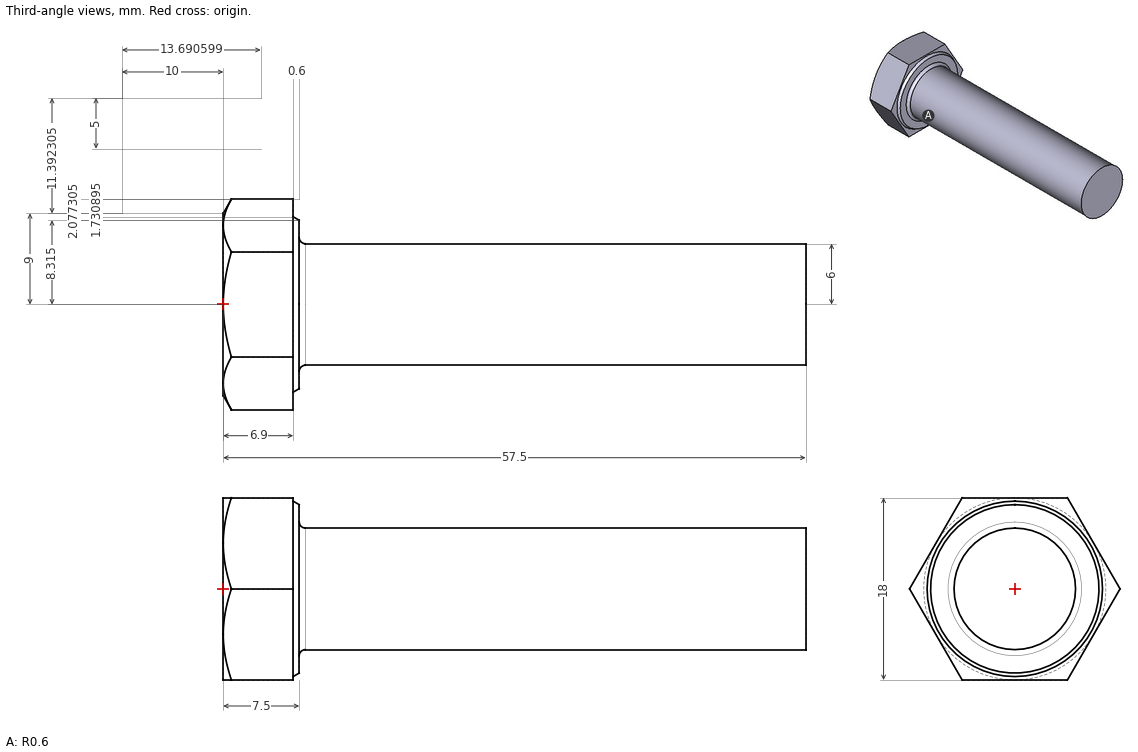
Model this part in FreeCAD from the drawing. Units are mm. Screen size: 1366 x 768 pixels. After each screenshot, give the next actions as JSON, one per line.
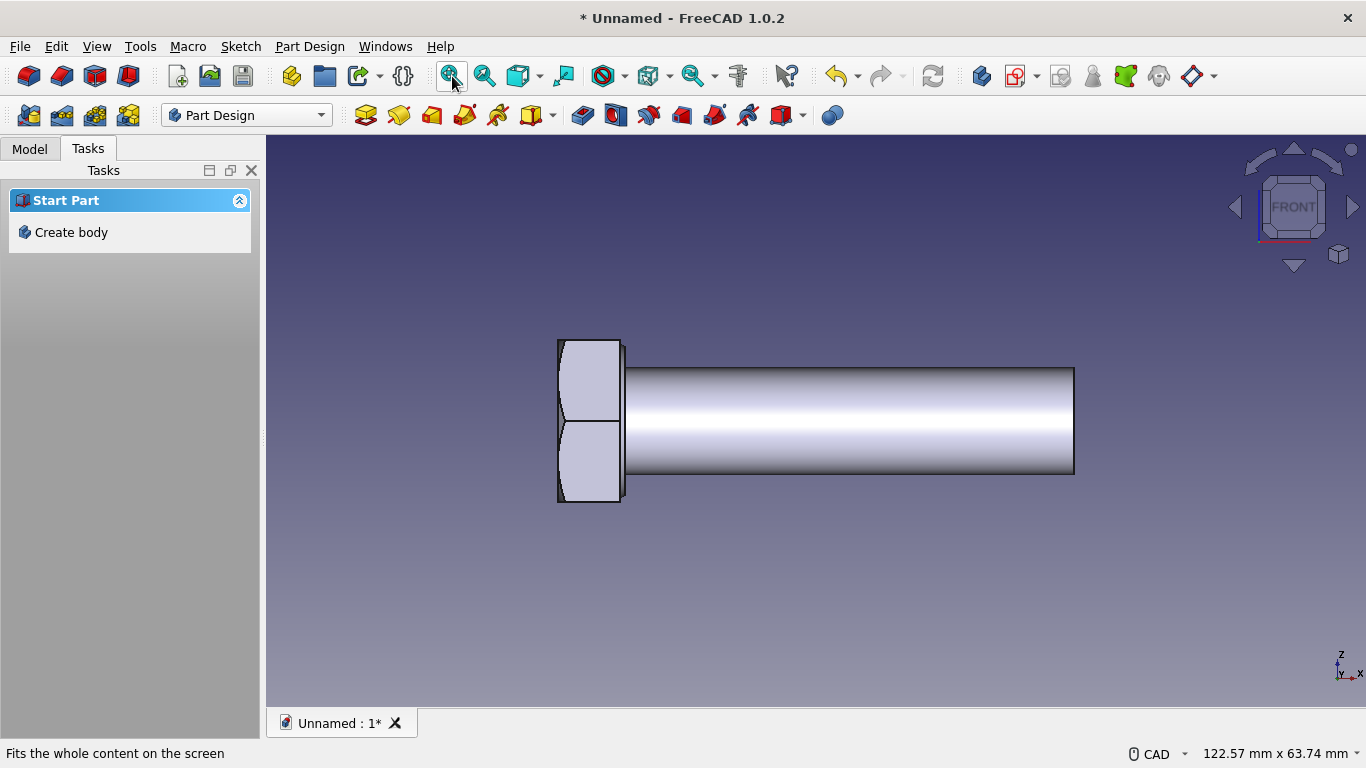
{"action": "key", "text": "3"}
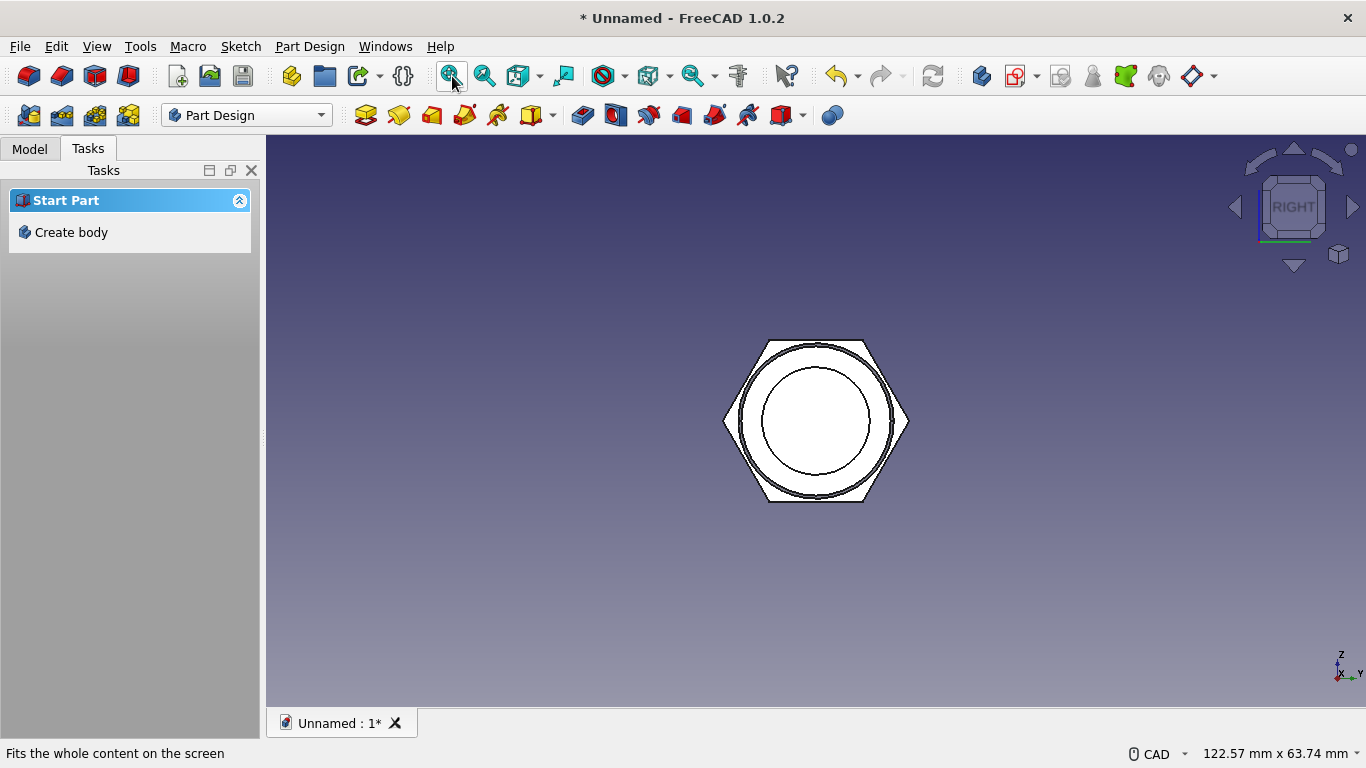
{"action": "left_click", "coordinate": [452, 76]}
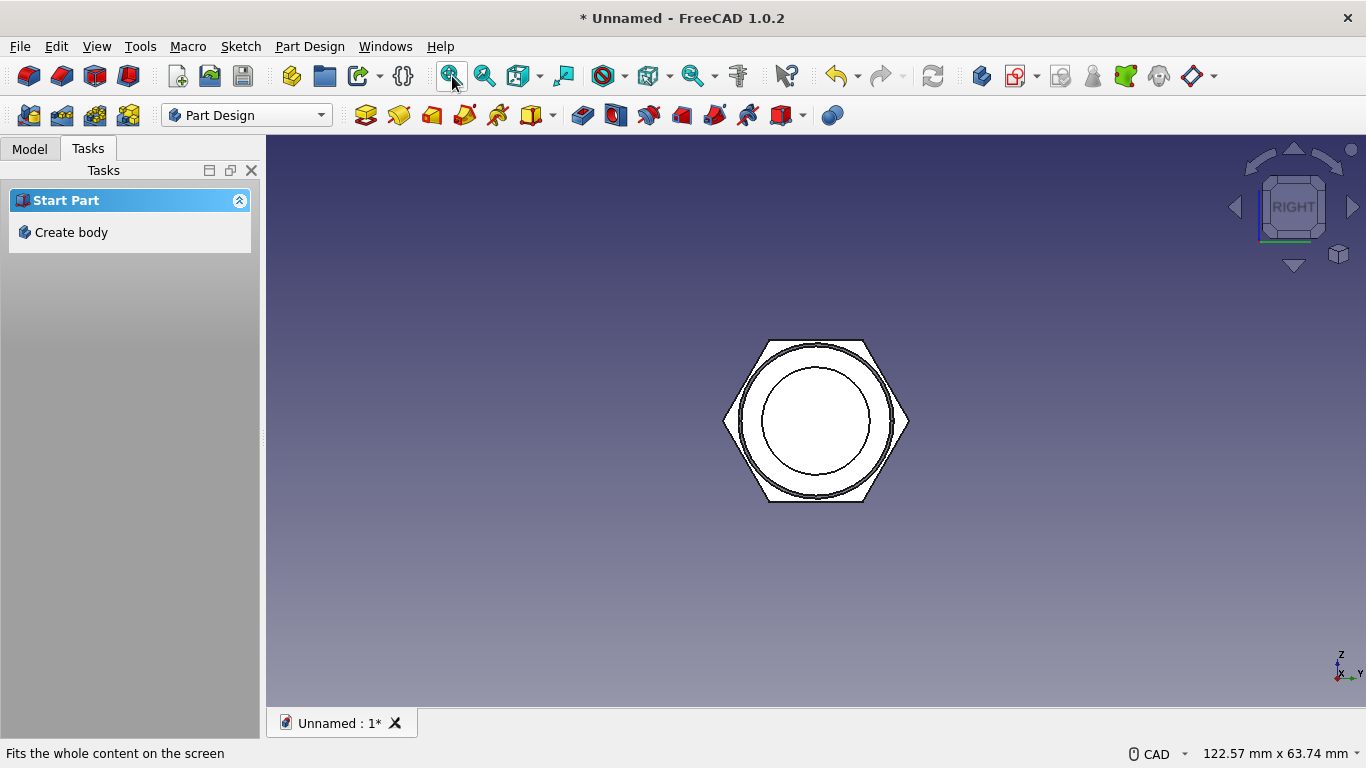
{"action": "key", "text": "5"}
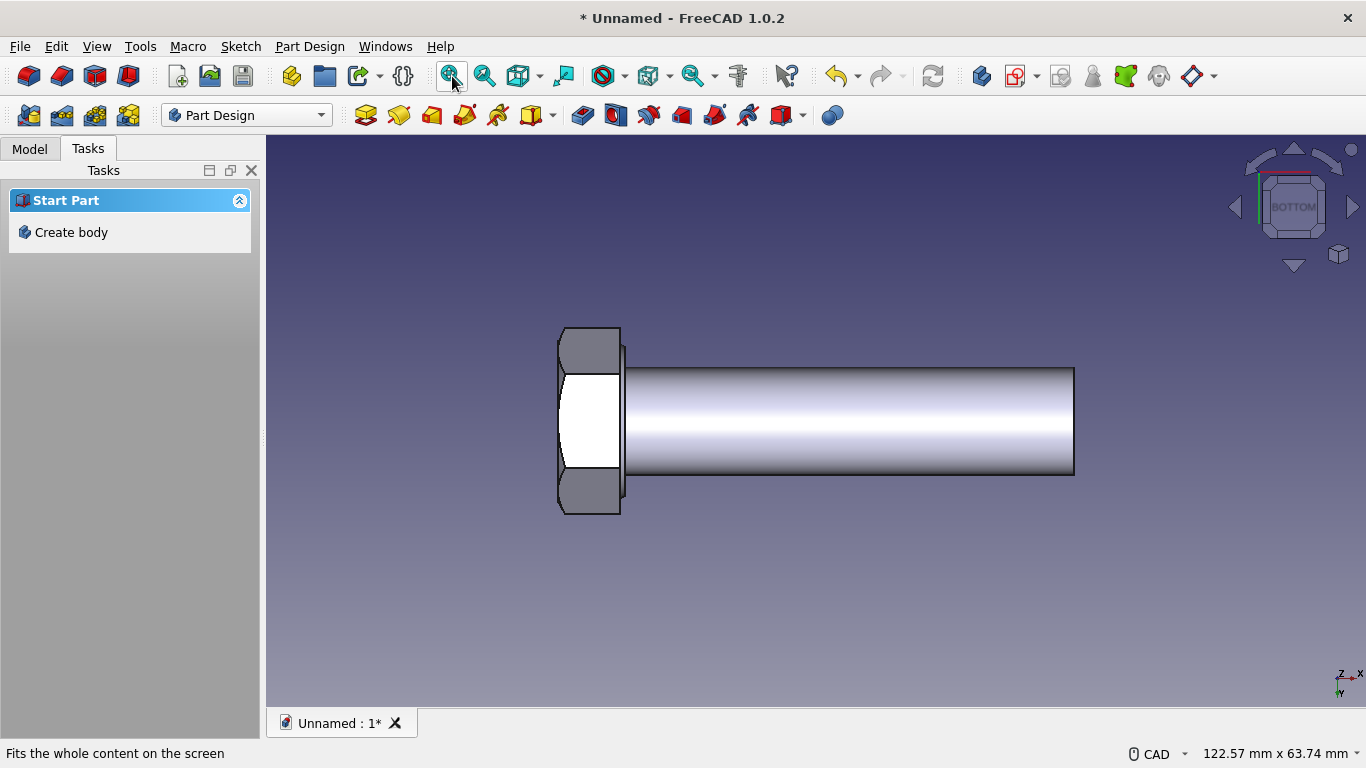
{"action": "key", "text": "4"}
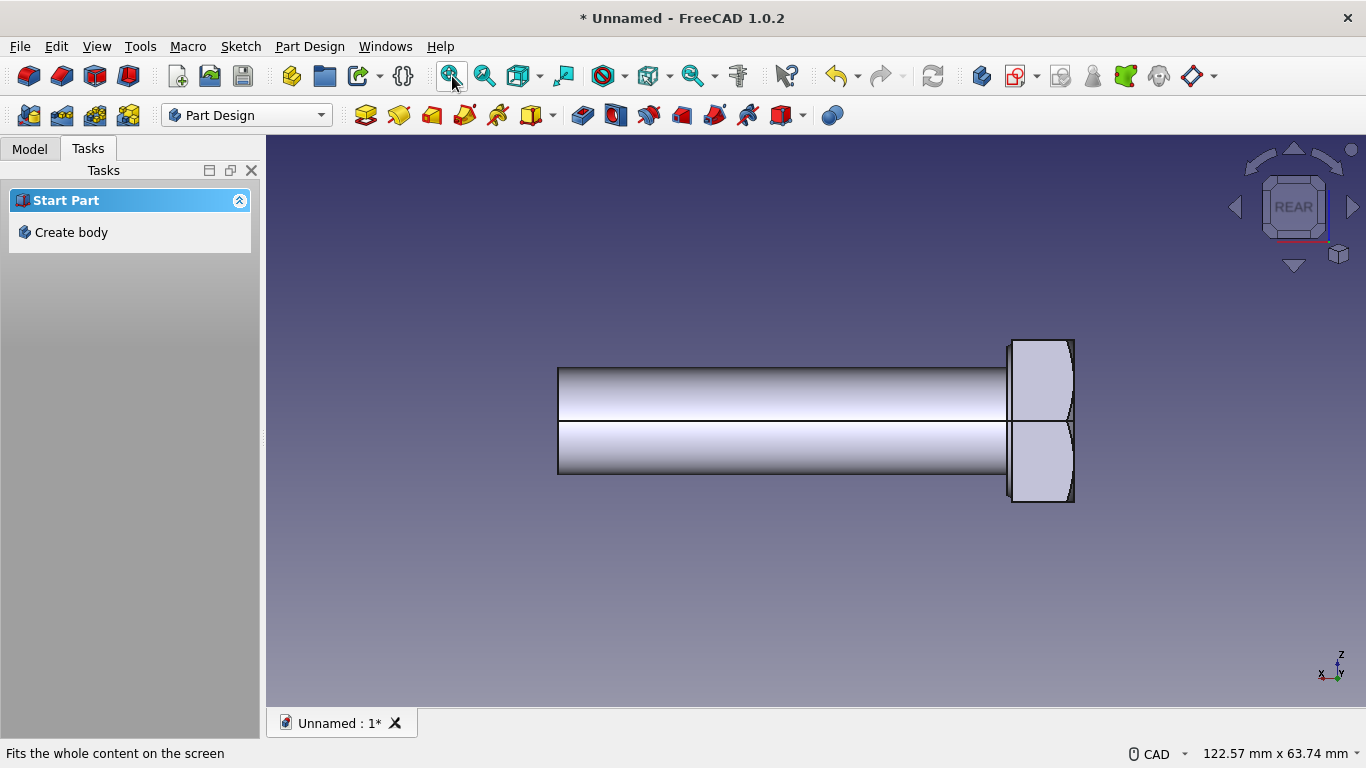
{"action": "key", "text": "6"}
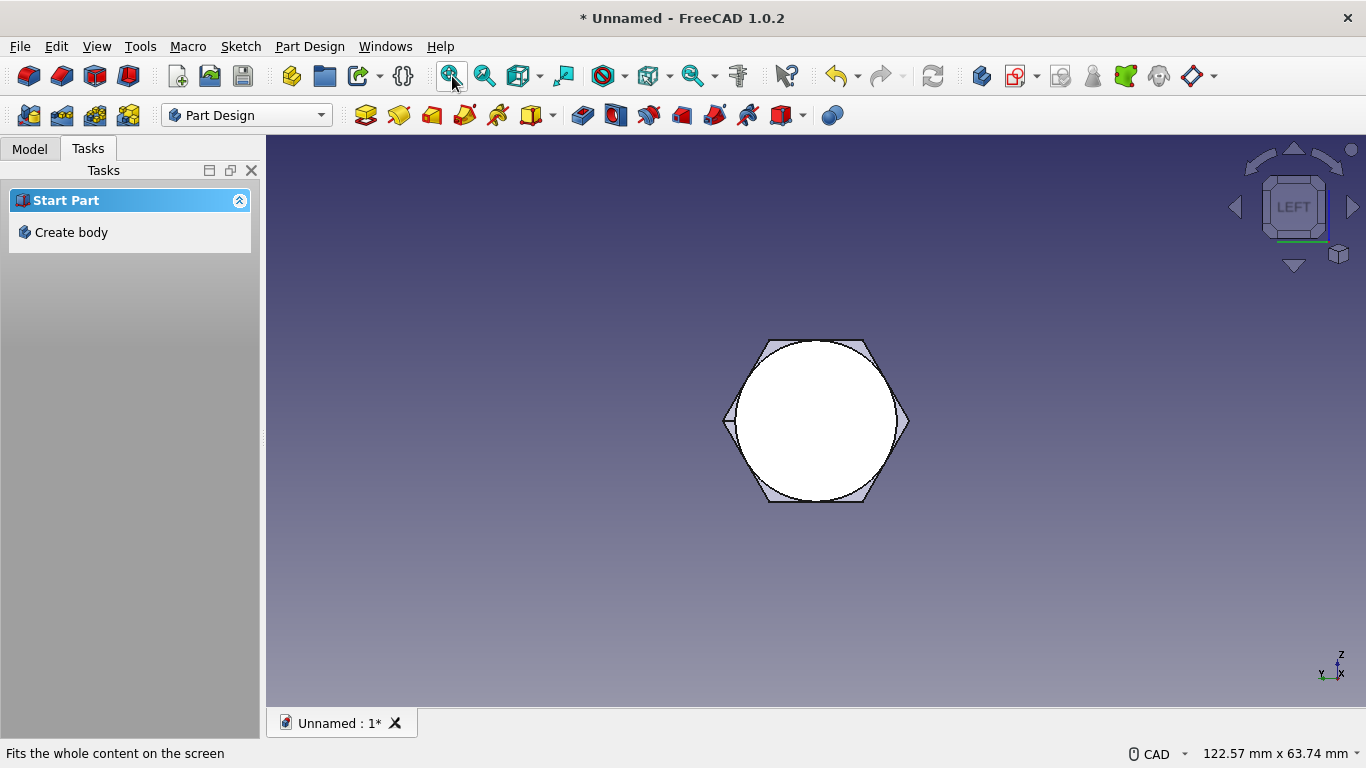
{"action": "key", "text": "v f"}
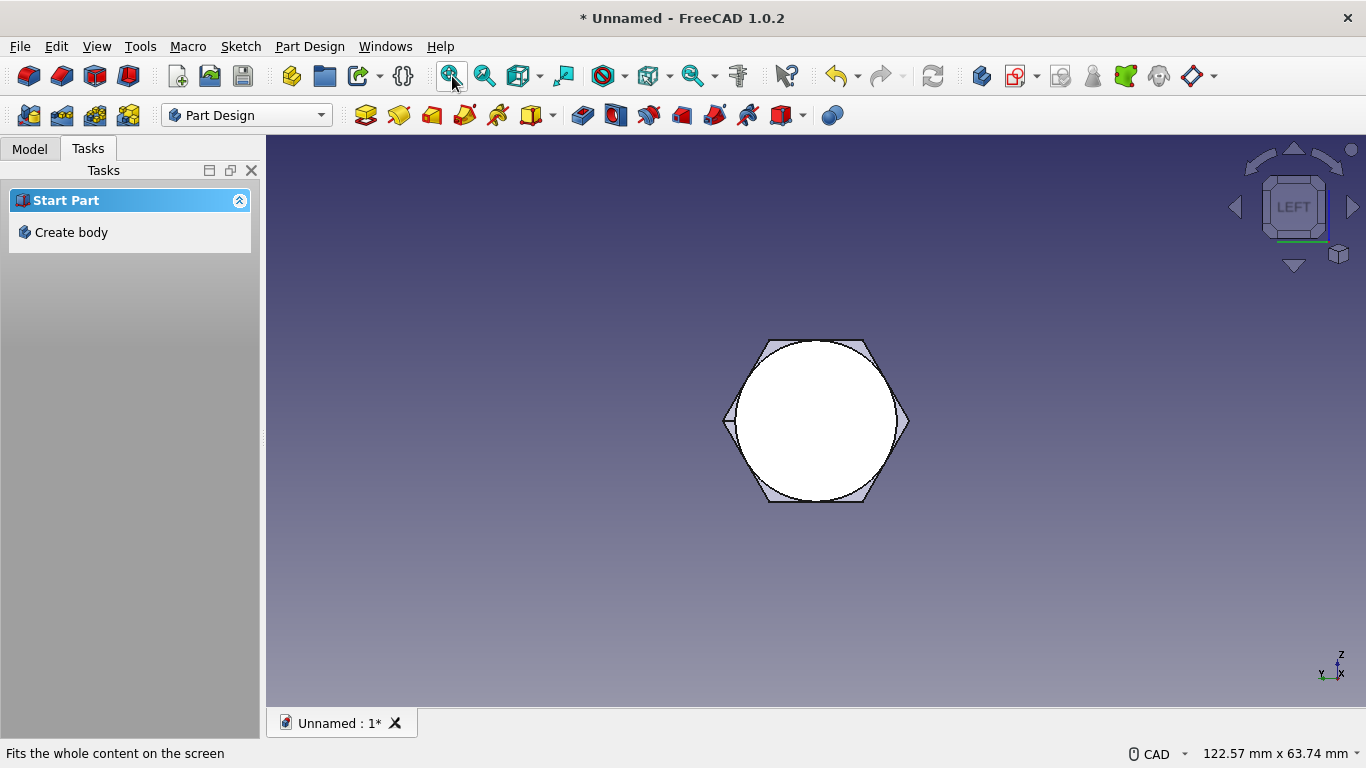
{"action": "key", "text": "v 3"}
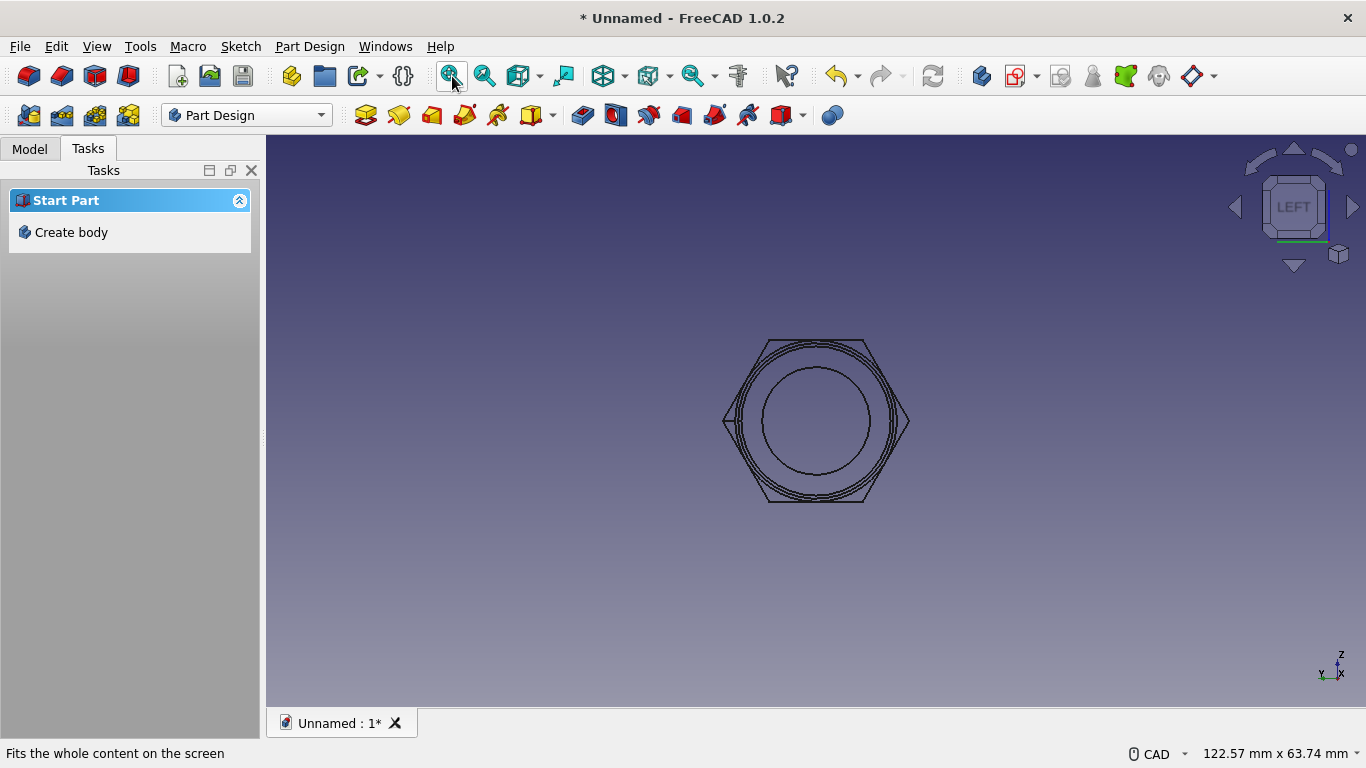
{"action": "key", "text": "0"}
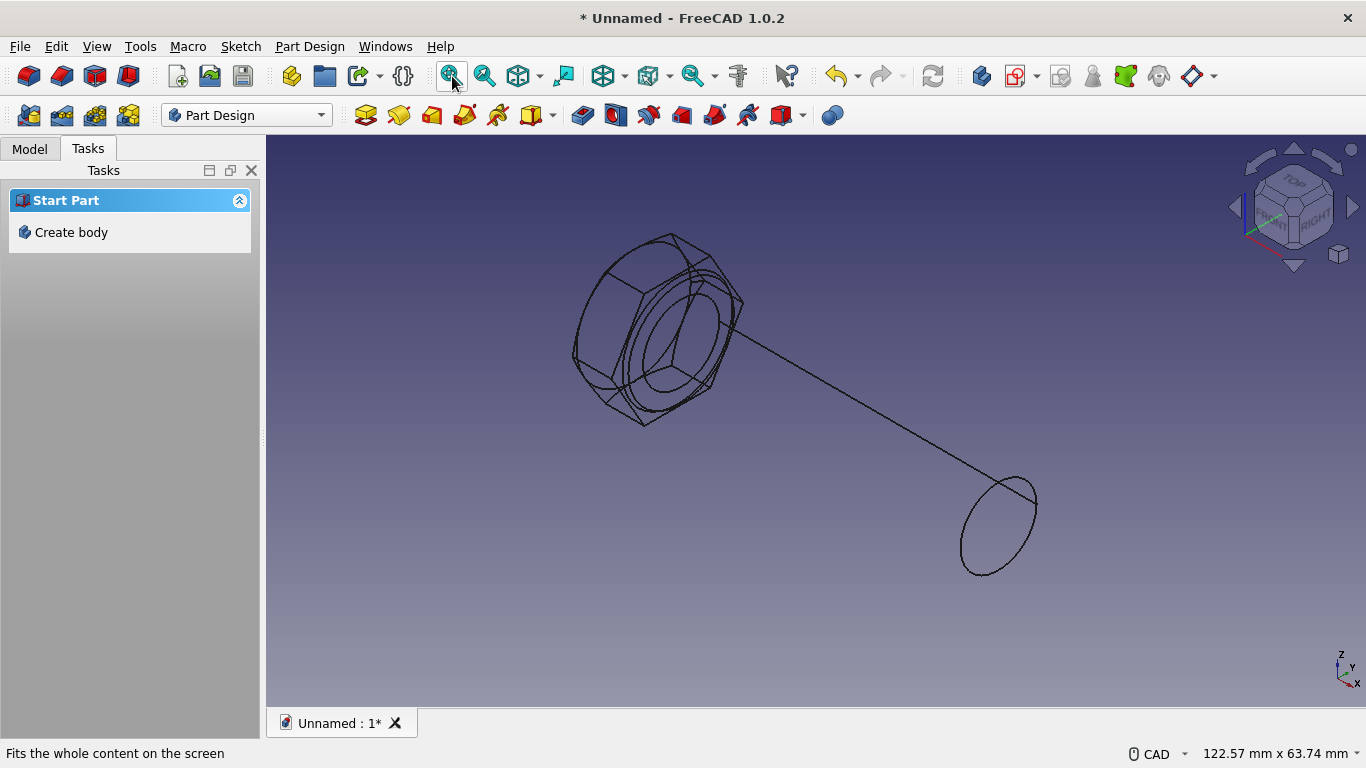
{"action": "left_click", "coordinate": [643, 364]}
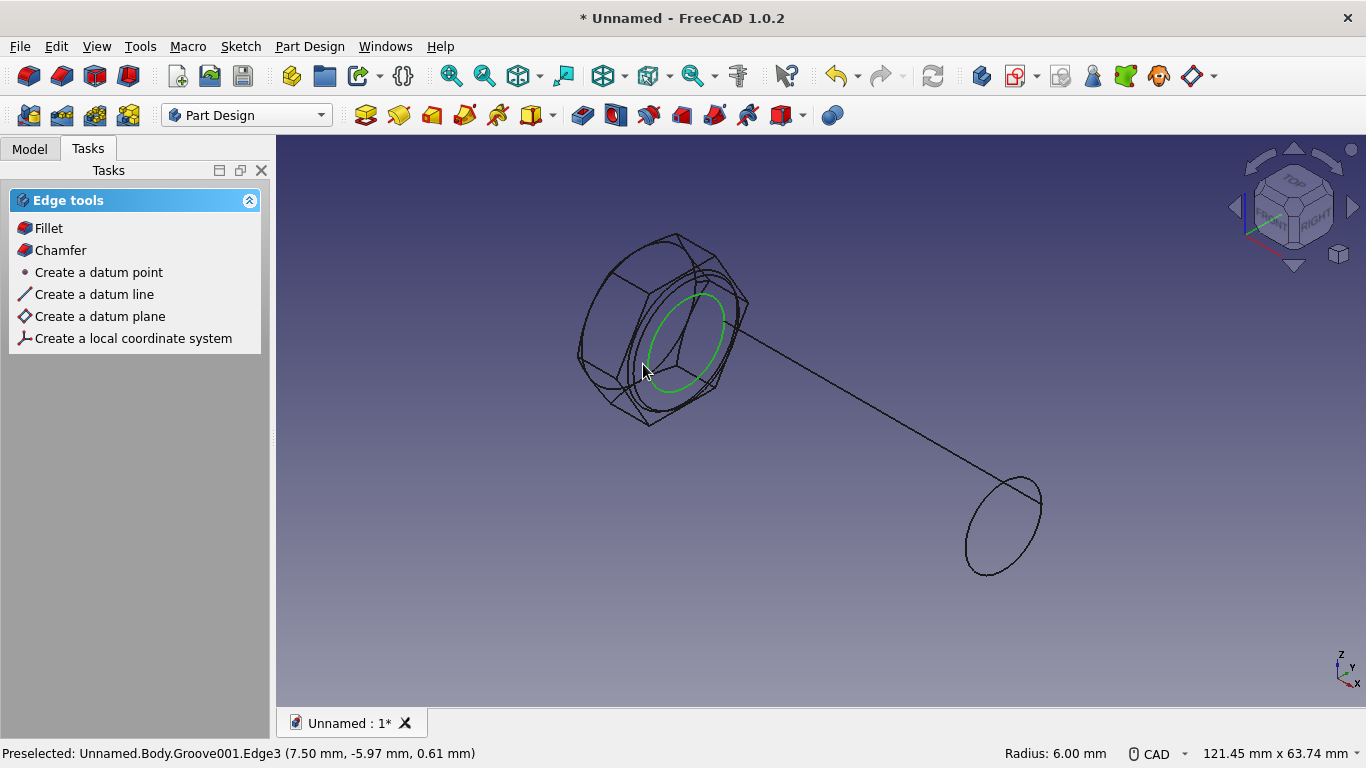
{"action": "key", "text": "v 1"}